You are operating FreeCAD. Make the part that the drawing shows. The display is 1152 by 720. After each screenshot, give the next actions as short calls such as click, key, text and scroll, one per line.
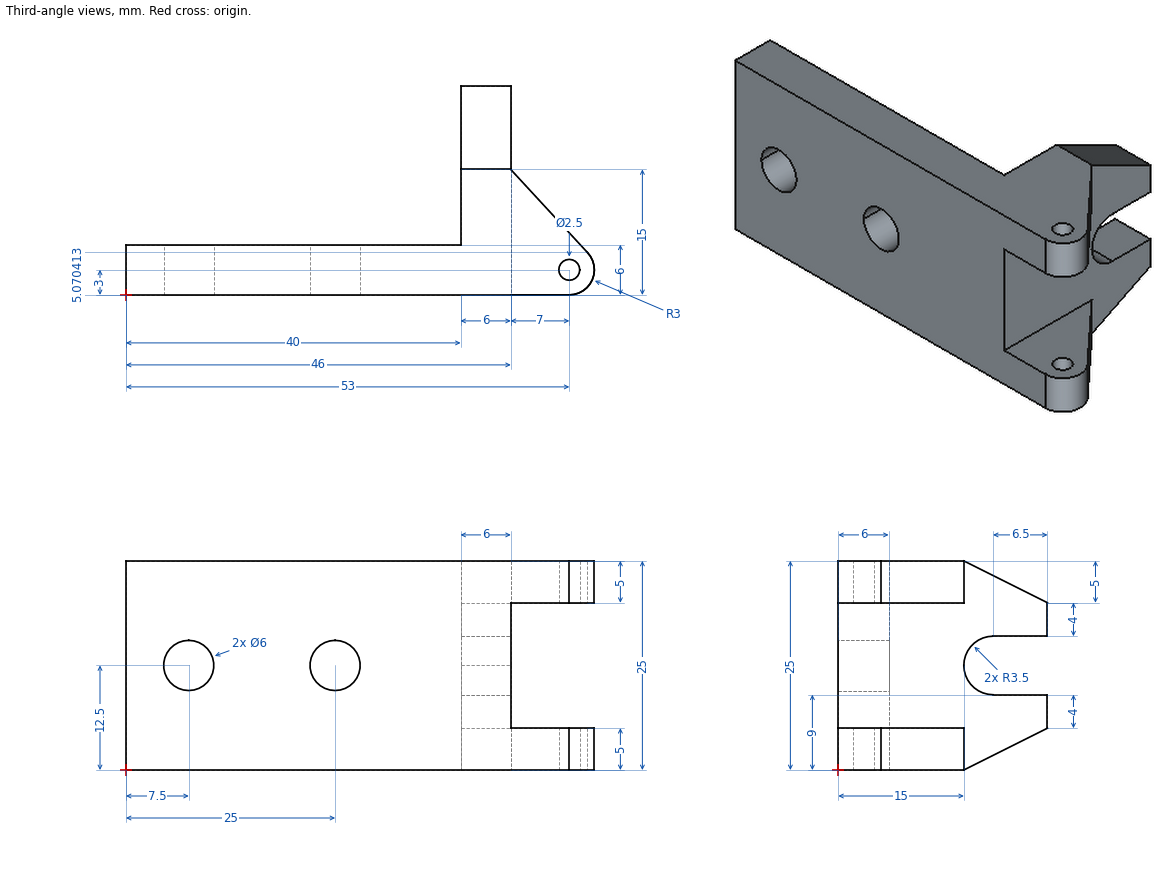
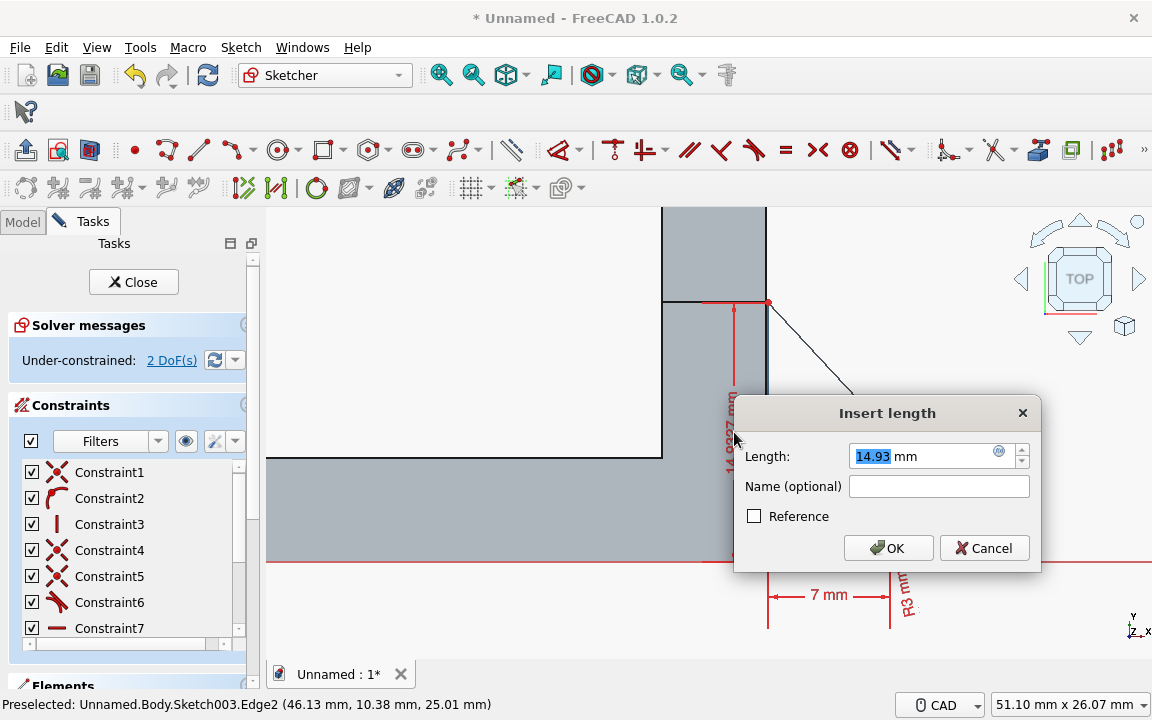
text(15)
key(Return)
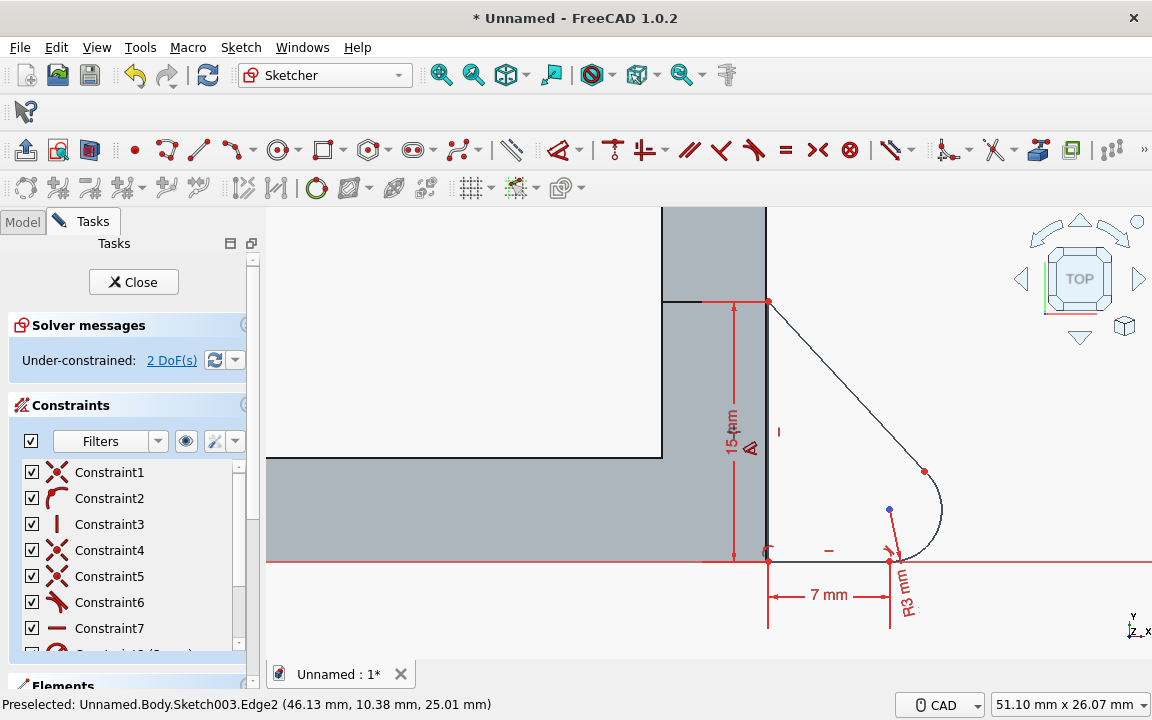
click(768, 302)
click(531, 596)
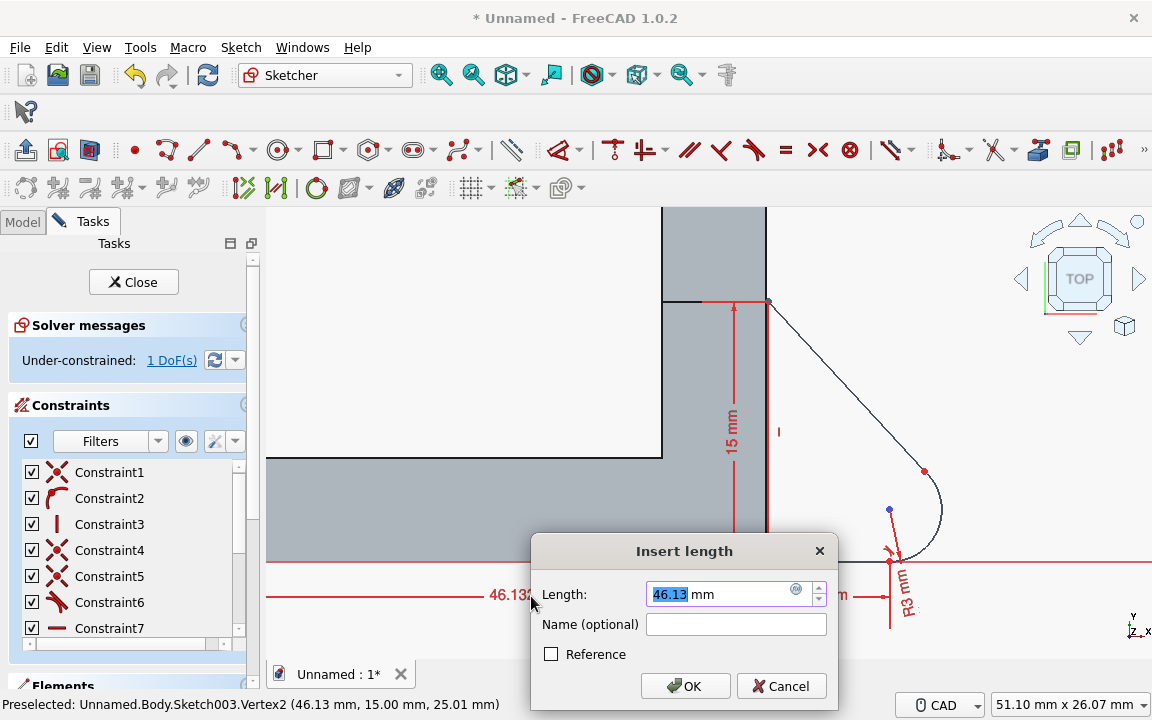
text(46)
key(Return)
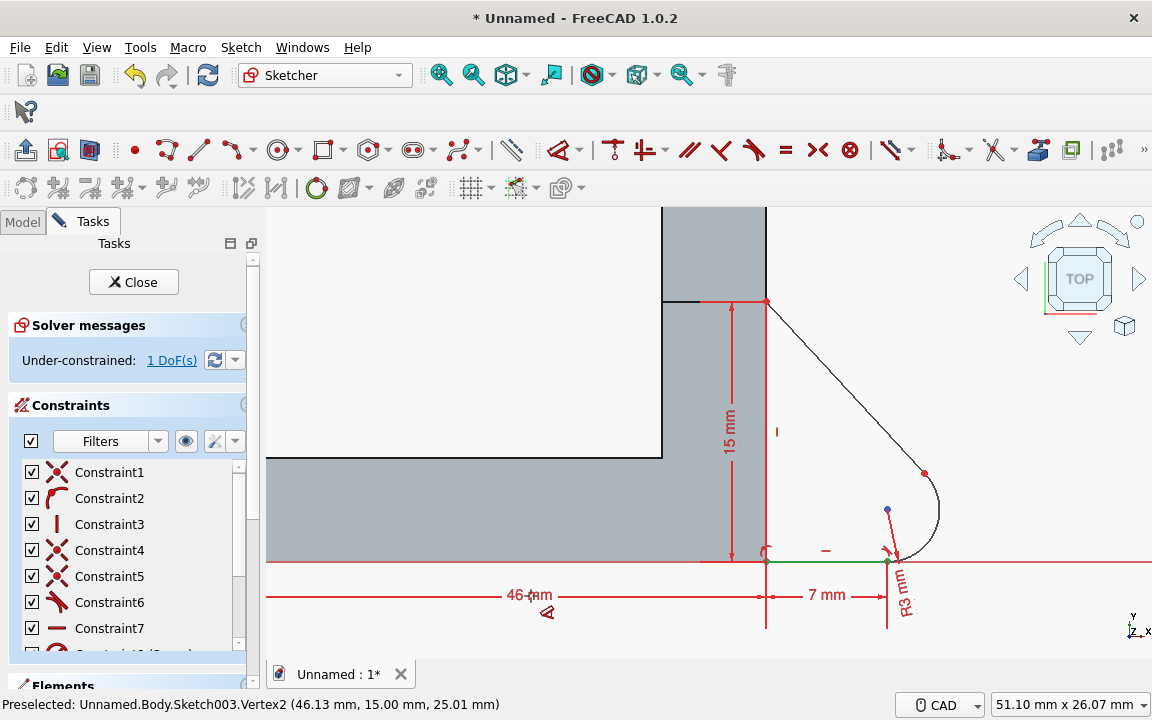
click(925, 474)
click(959, 518)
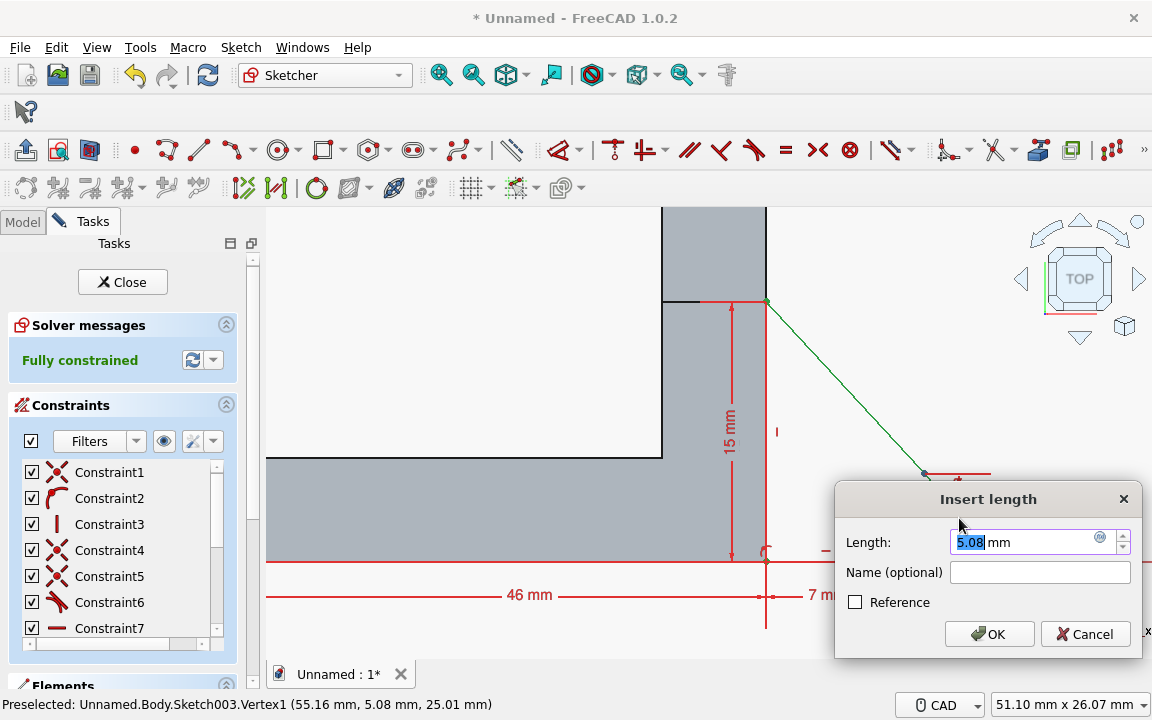
text(5.070413)
key(Return)
key(Escape)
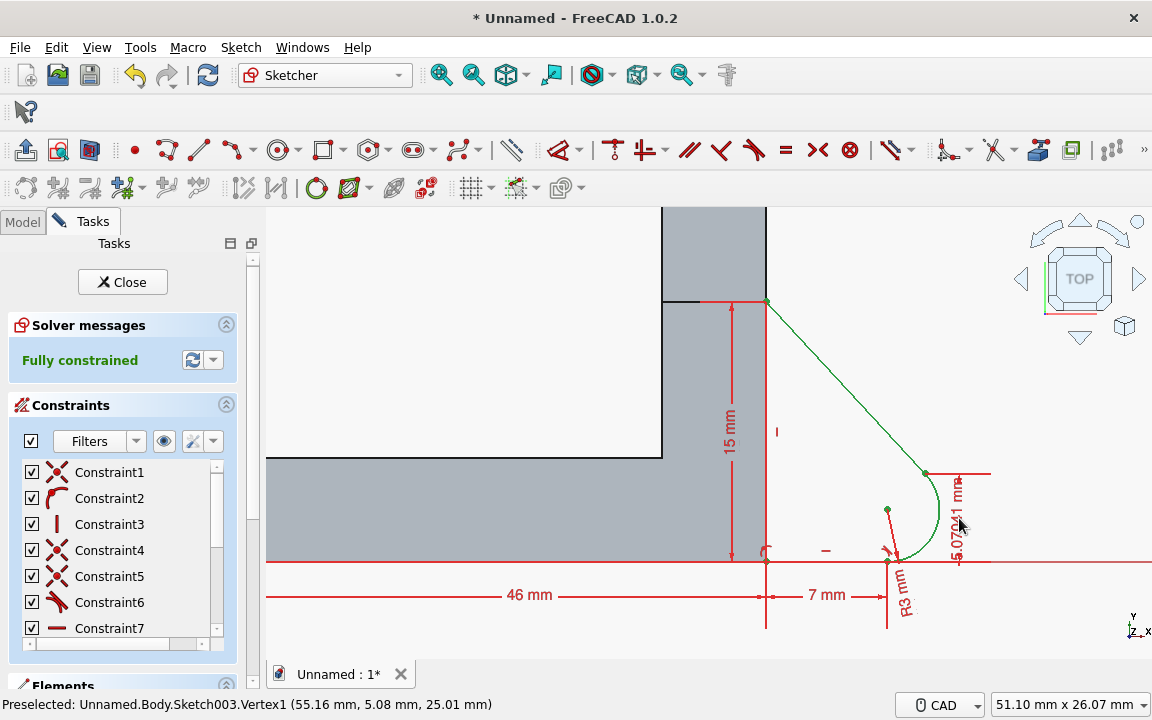
click(123, 282)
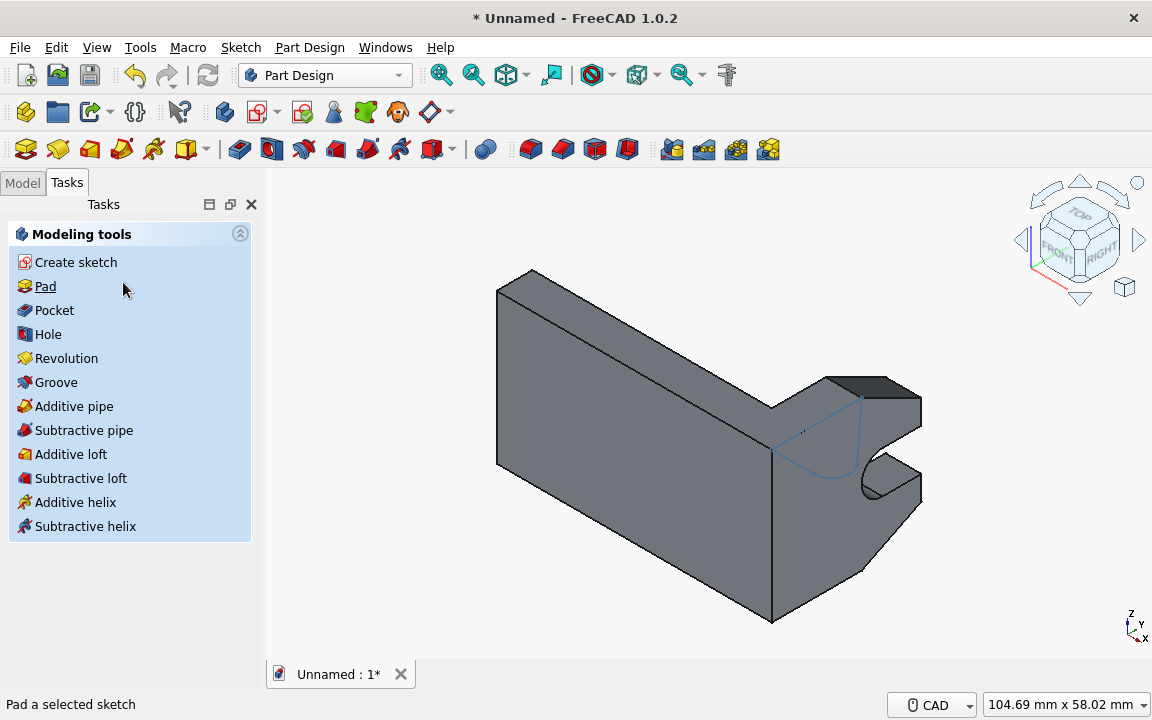
click(26, 150)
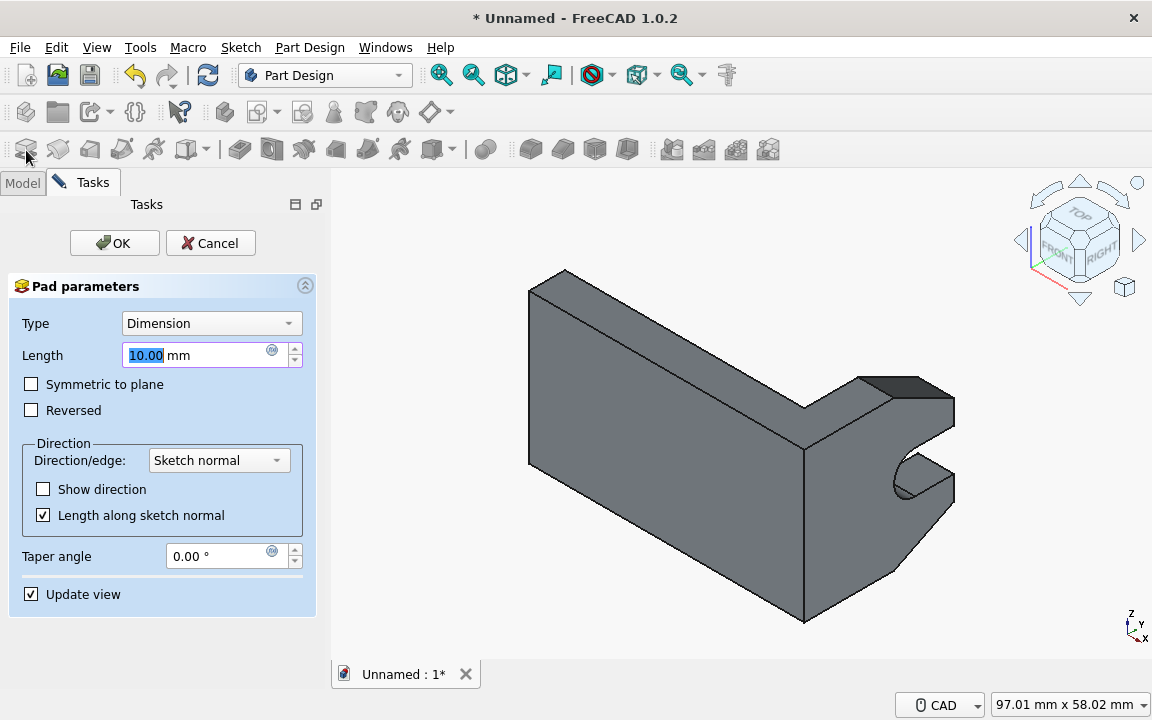
text(5)
key(Tab)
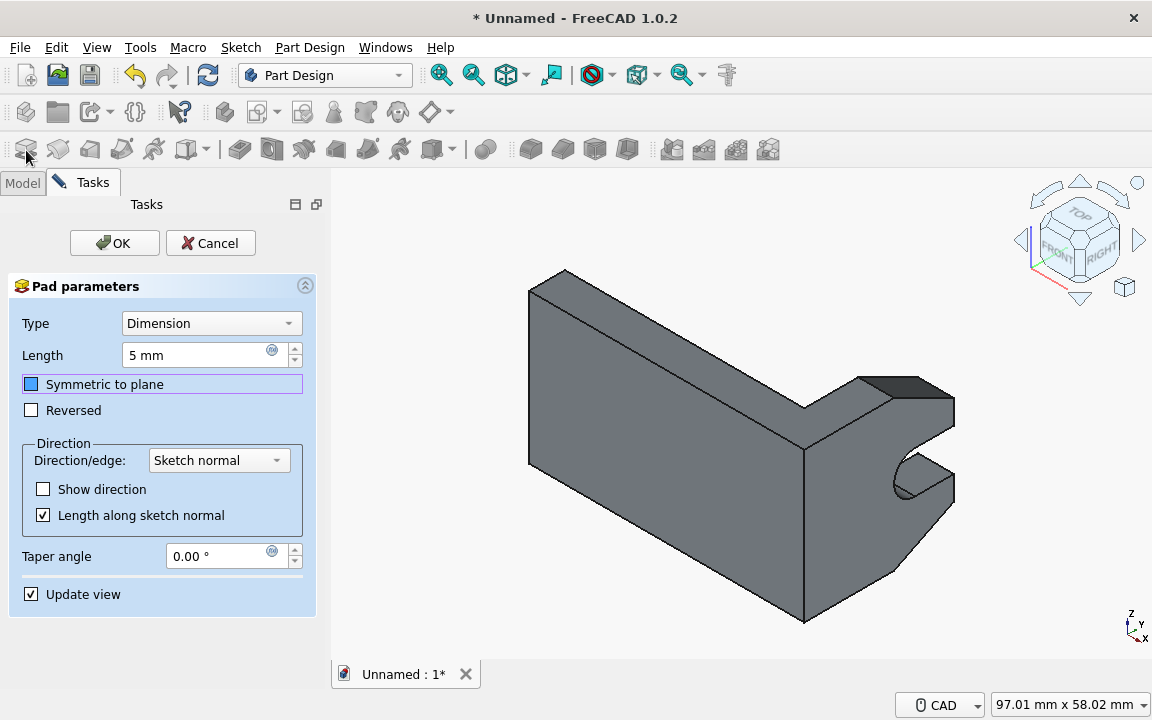
click(30, 410)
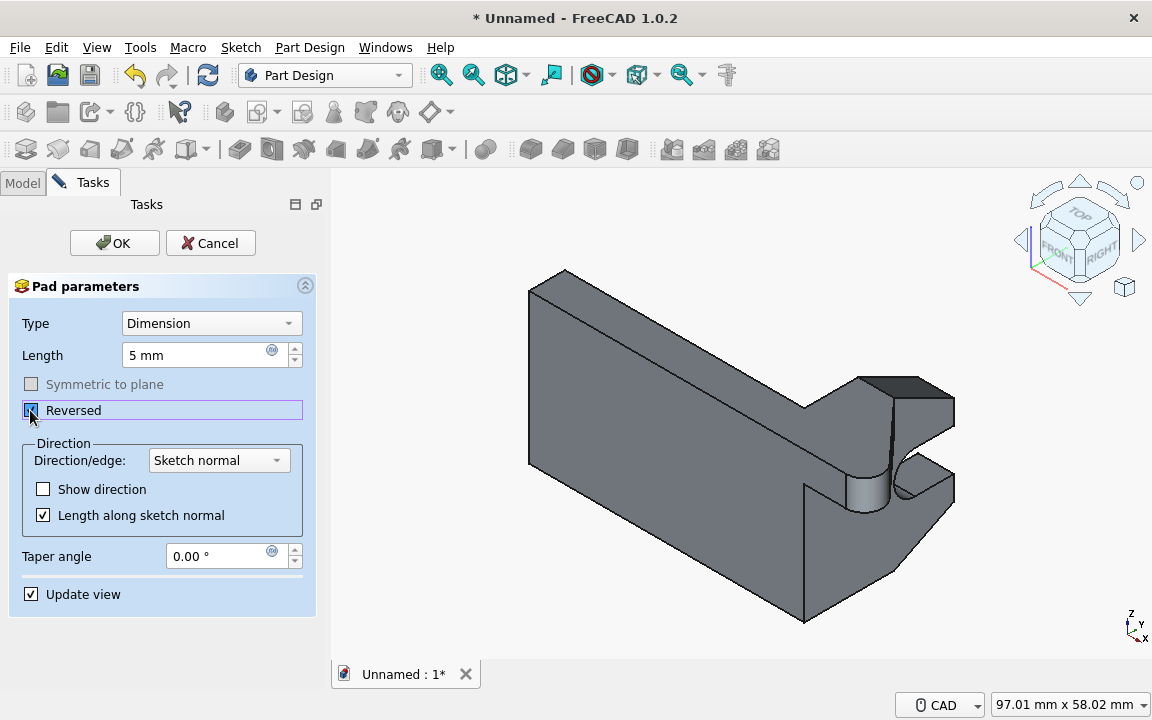
click(115, 243)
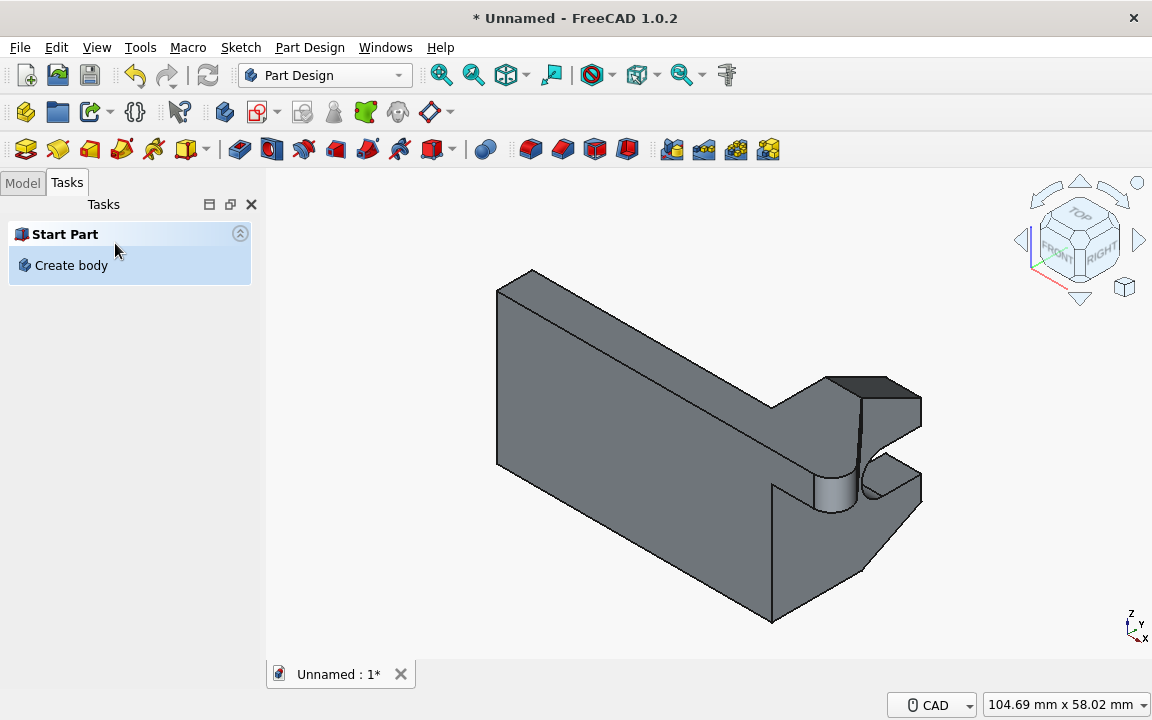
click(792, 423)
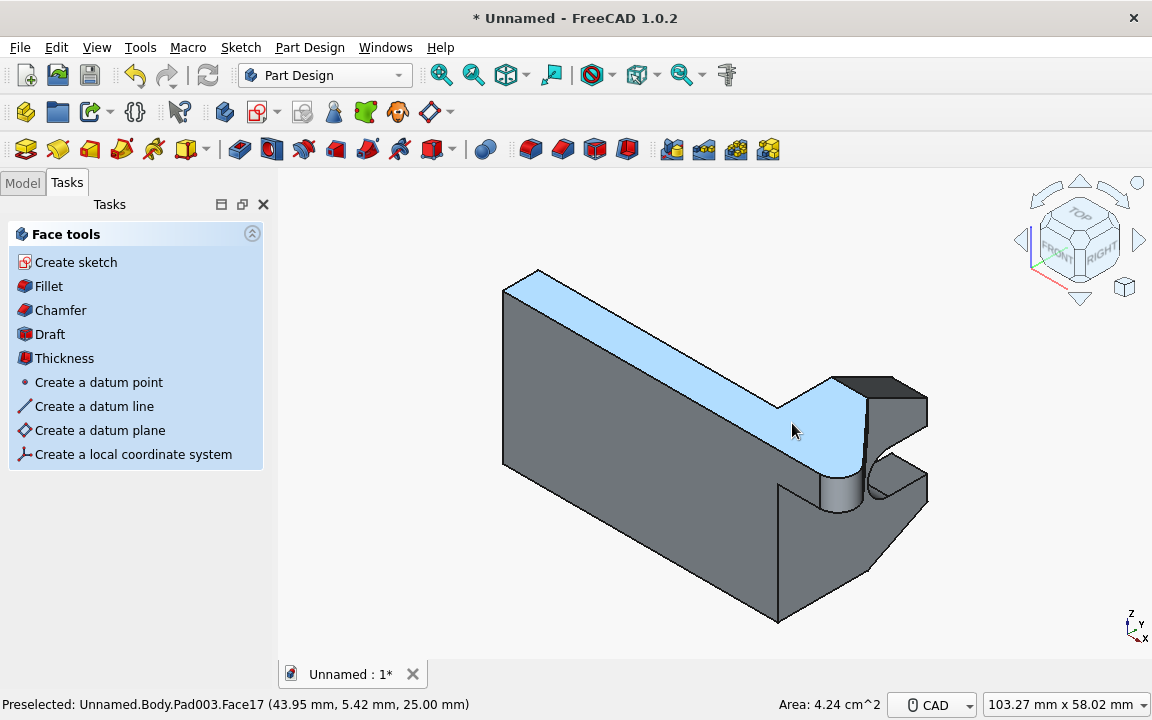
click(258, 112)